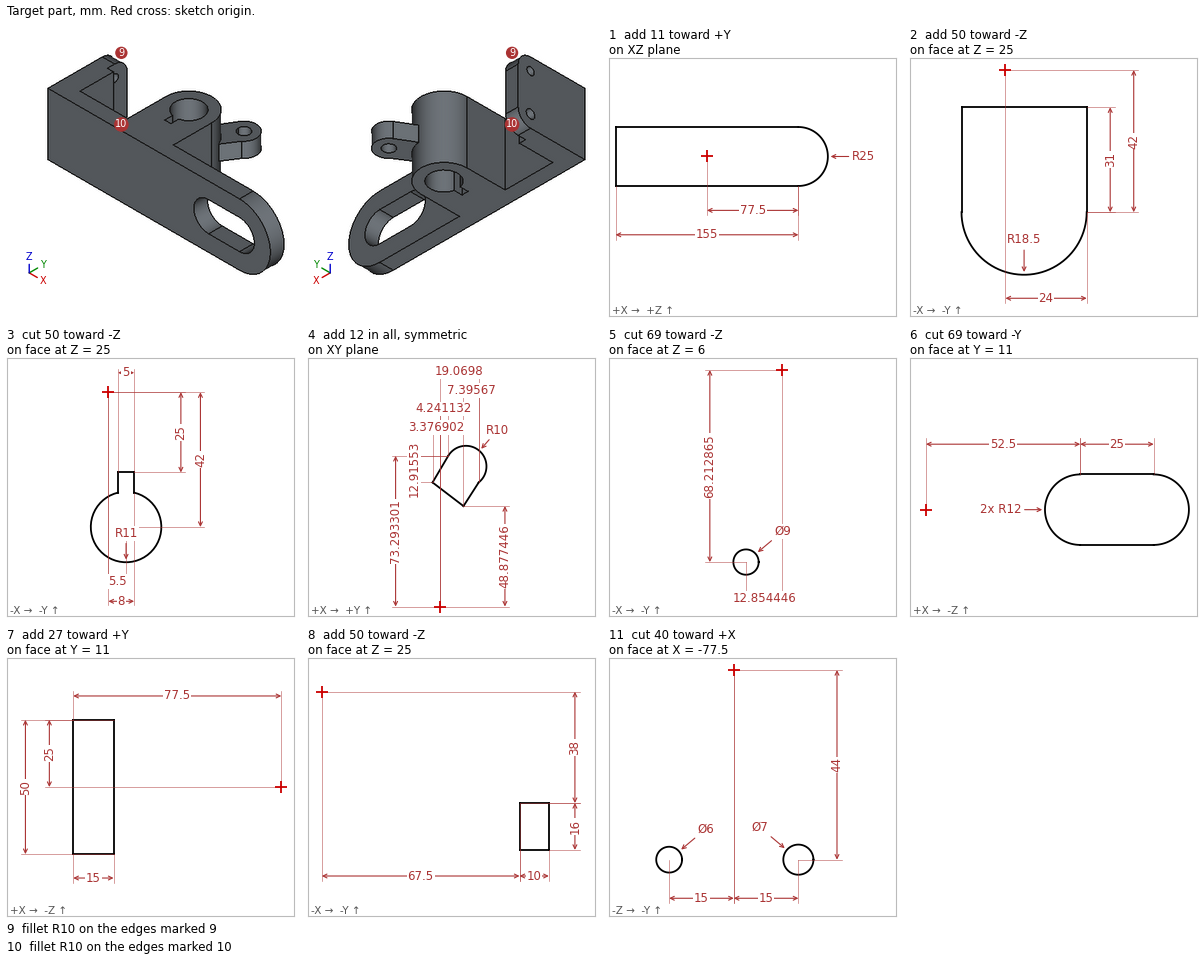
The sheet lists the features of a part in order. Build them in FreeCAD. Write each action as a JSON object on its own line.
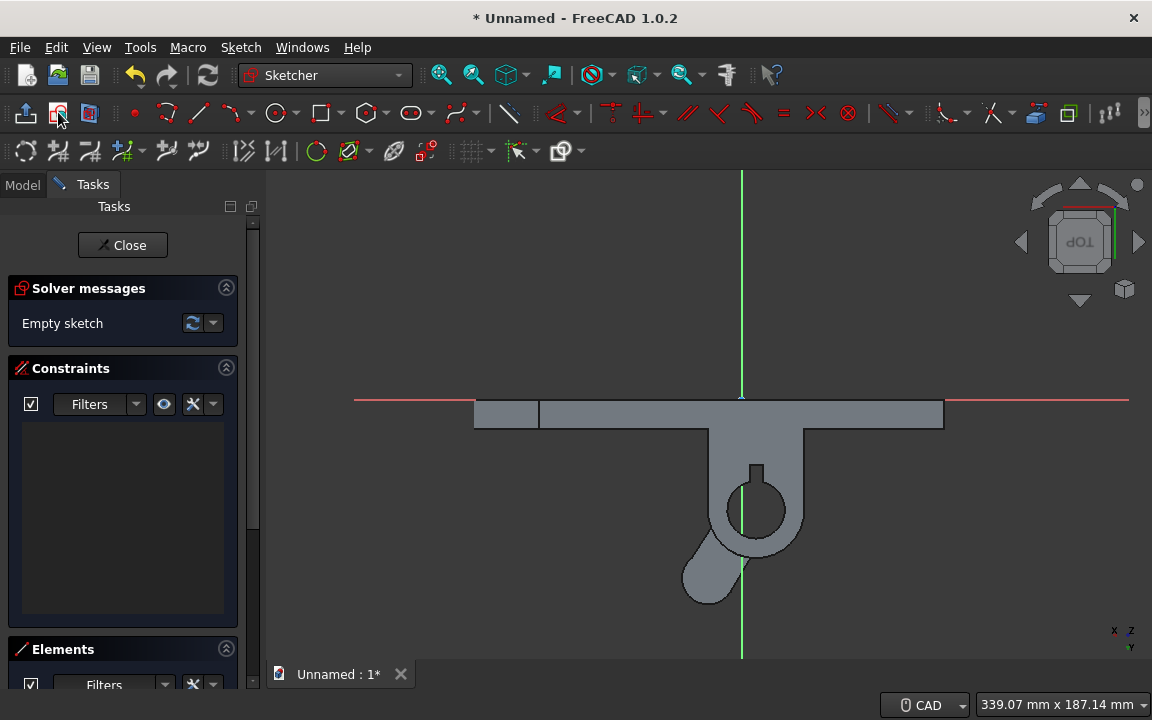
{"action": "left_click", "coordinate": [90, 114]}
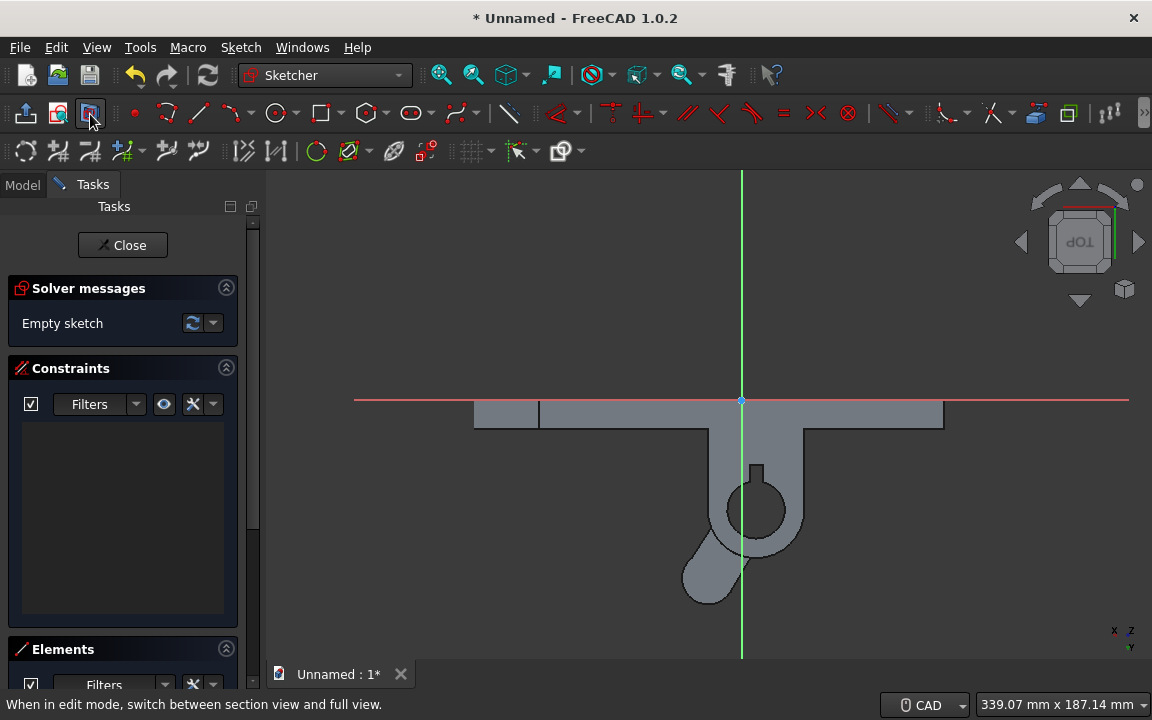
{"action": "scroll", "coordinate": [713, 592], "scroll_direction": "up", "scroll_amount": 13}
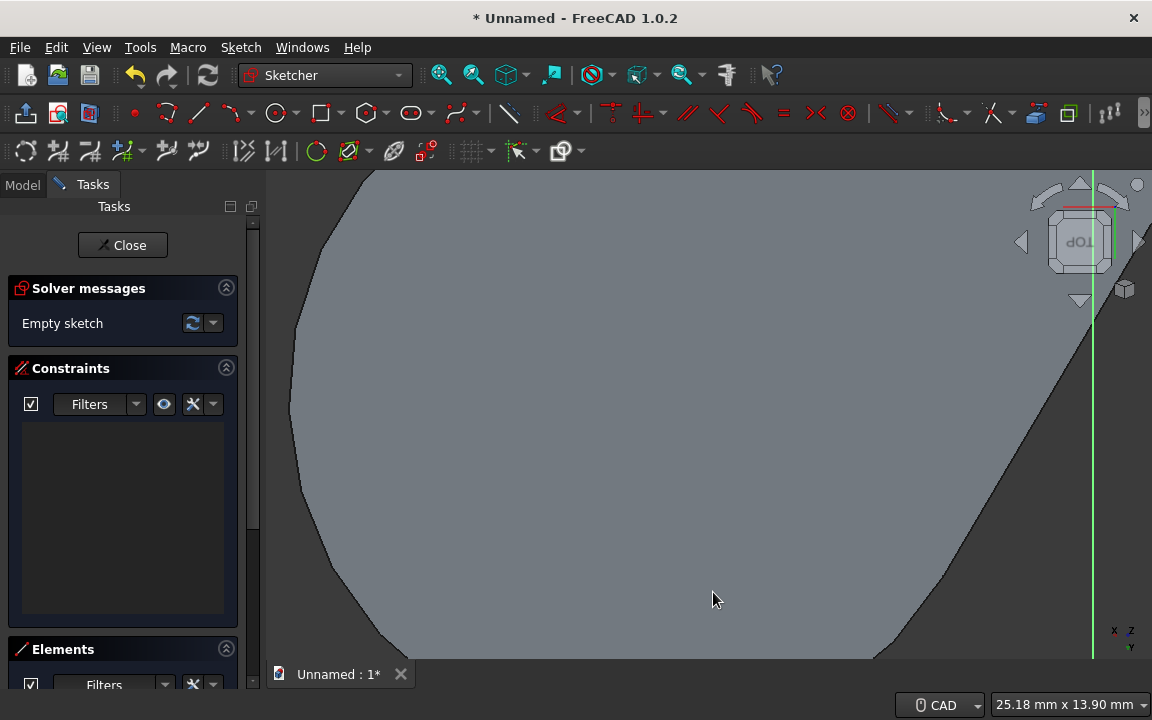
{"action": "left_click", "coordinate": [276, 114]}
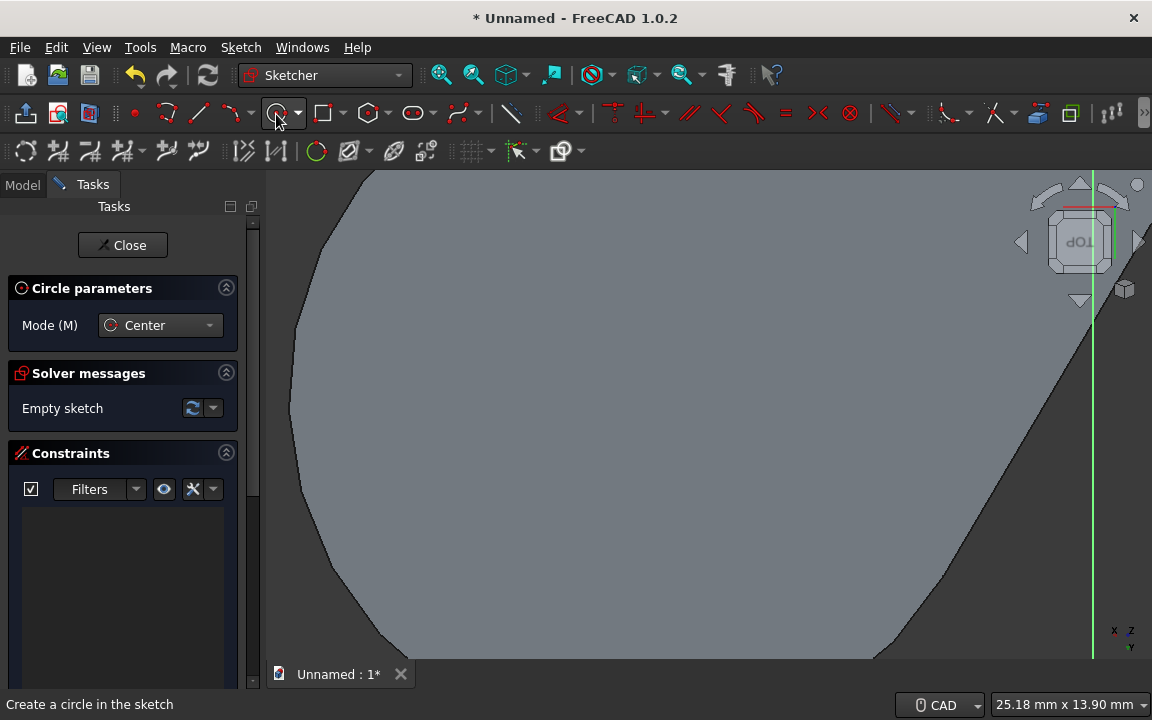
{"action": "left_click", "coordinate": [640, 398]}
{"action": "mouse_move", "coordinate": [752, 286]}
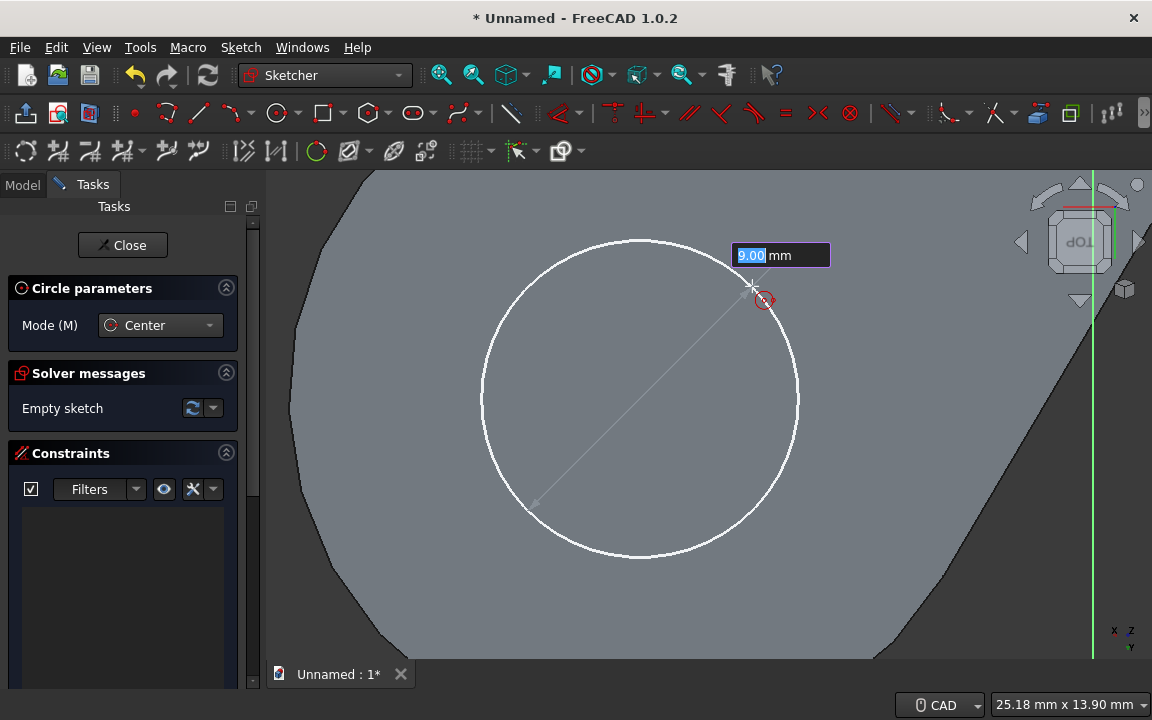
{"action": "type", "text": "9"}
{"action": "key", "text": "Return"}
{"action": "key", "text": "Escape"}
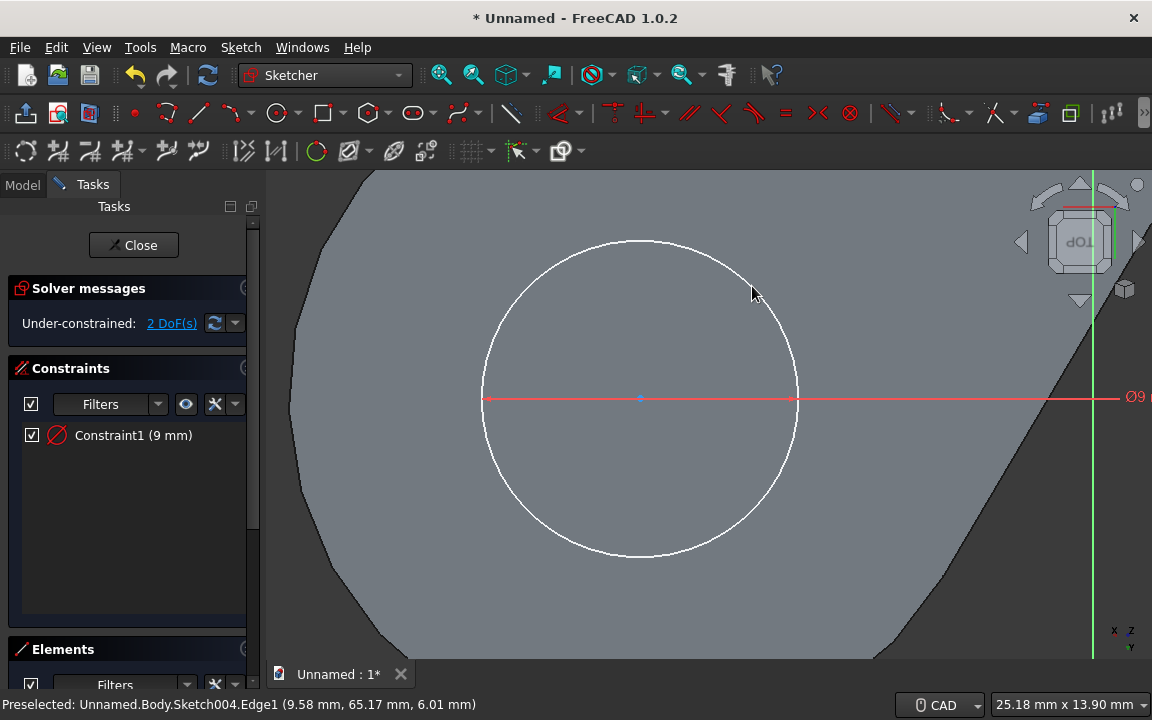
{"action": "left_click", "coordinate": [558, 114]}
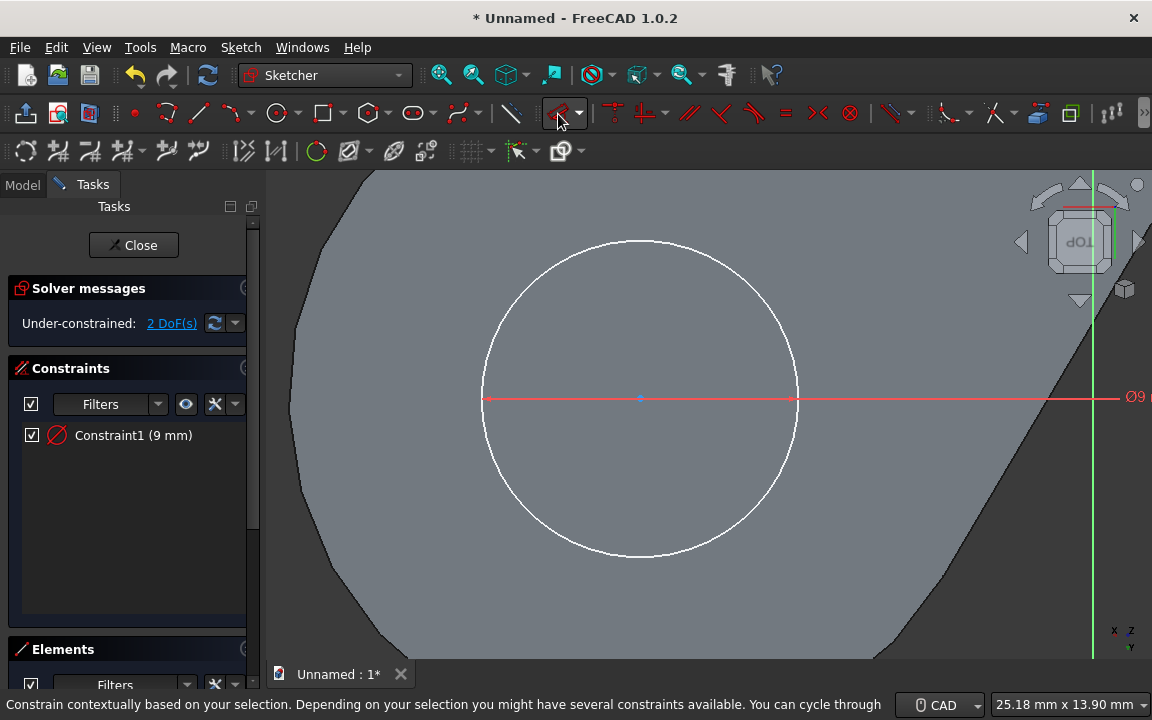
{"action": "left_click", "coordinate": [640, 399]}
{"action": "left_click", "coordinate": [814, 433]}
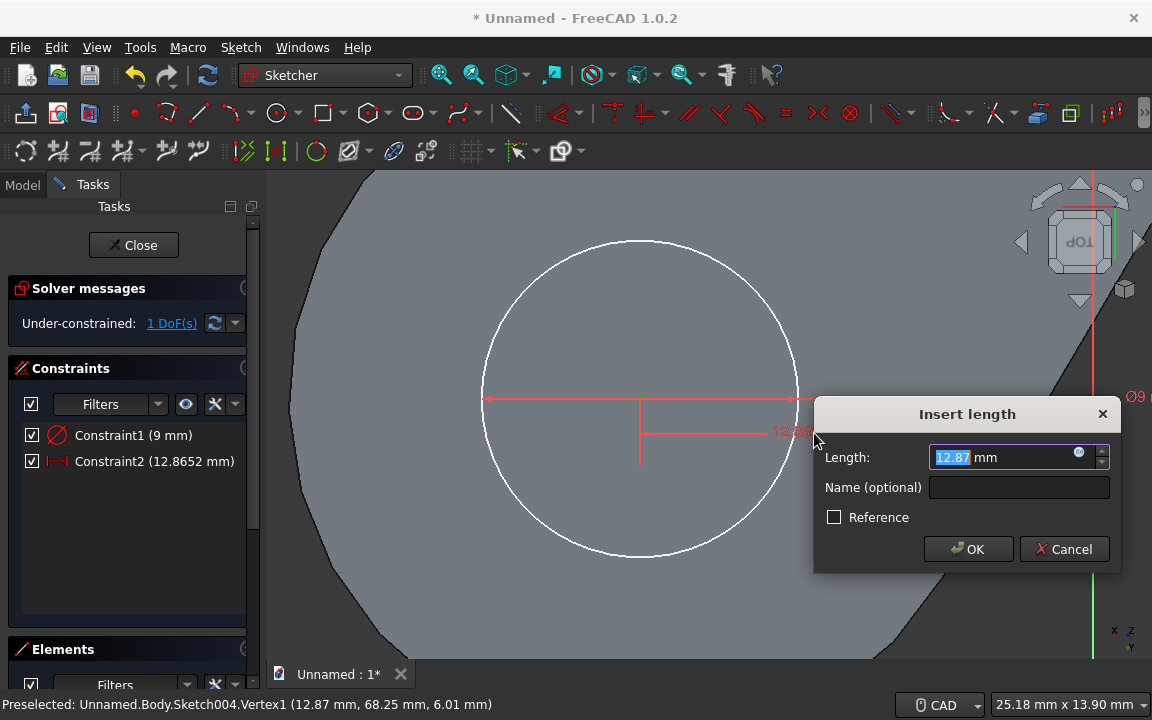
{"action": "type", "text": "12.854446"}
{"action": "key", "text": "Return"}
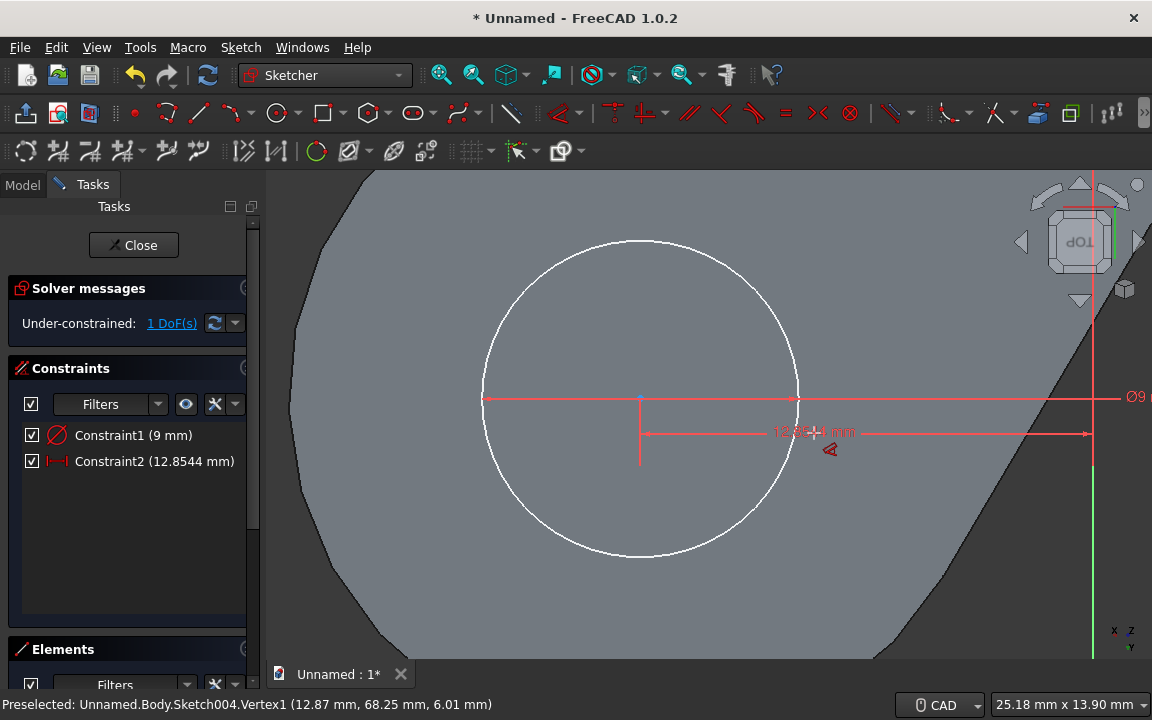
{"action": "left_click", "coordinate": [640, 399]}
{"action": "left_click", "coordinate": [606, 299]}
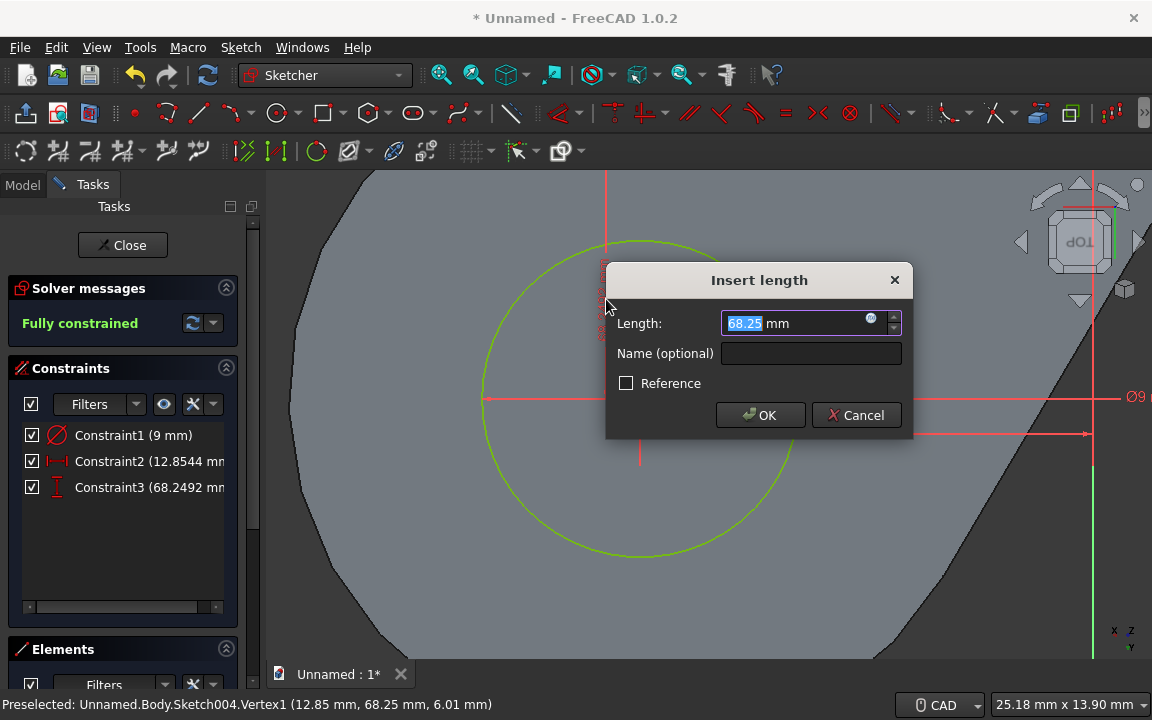
{"action": "type", "text": "68.212865"}
{"action": "key", "text": "Return"}
{"action": "key", "text": "Escape"}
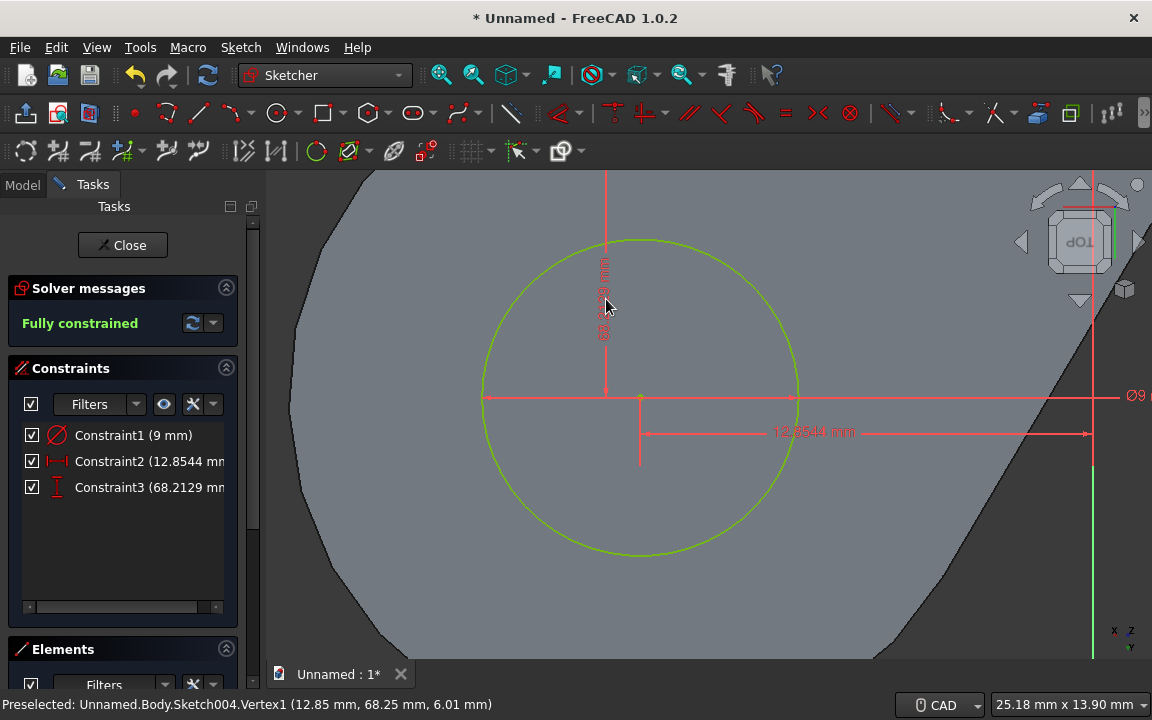
{"action": "left_click", "coordinate": [123, 245]}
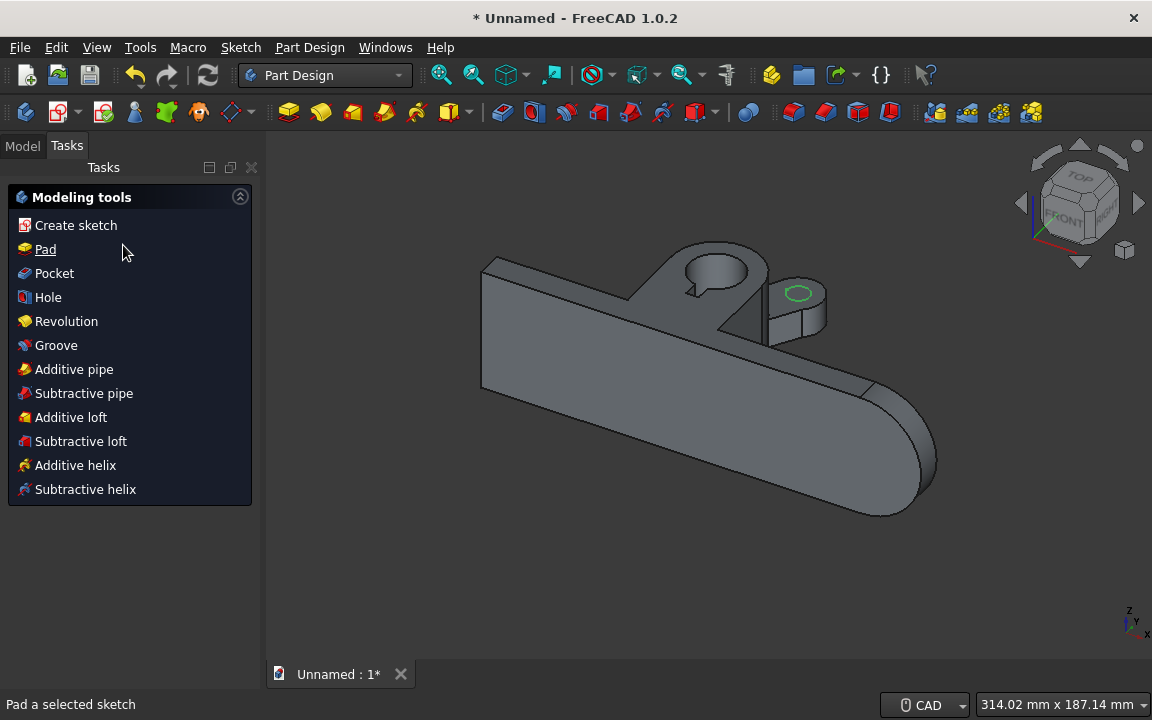
{"action": "left_click", "coordinate": [504, 112]}